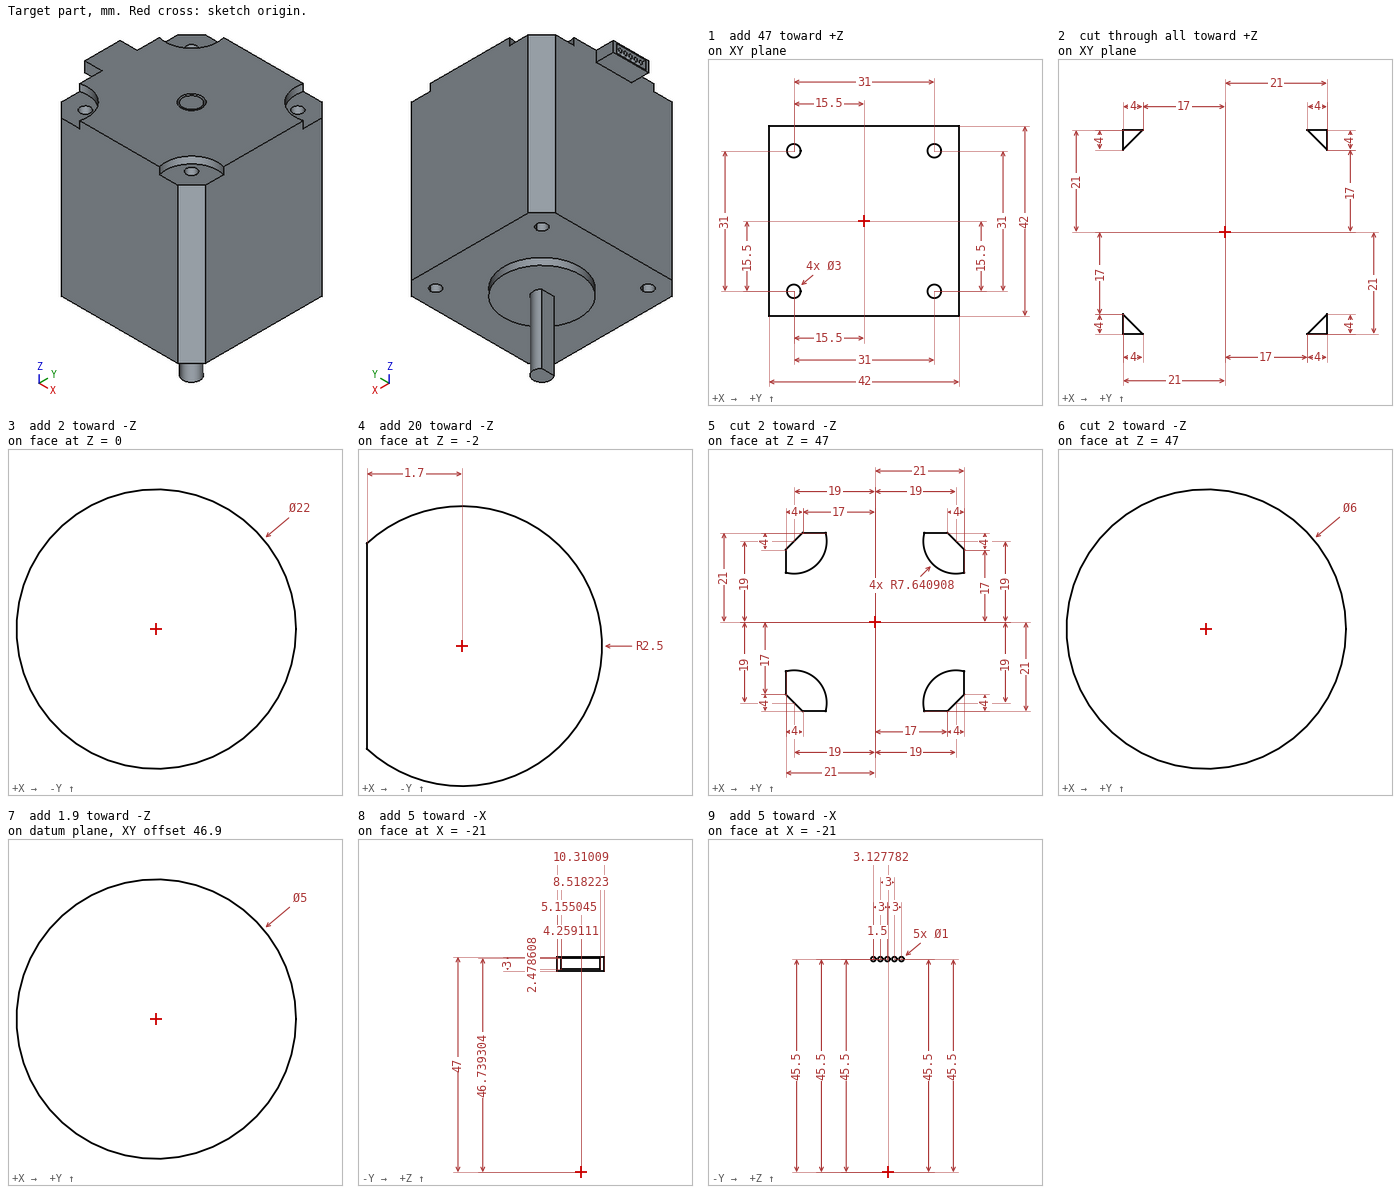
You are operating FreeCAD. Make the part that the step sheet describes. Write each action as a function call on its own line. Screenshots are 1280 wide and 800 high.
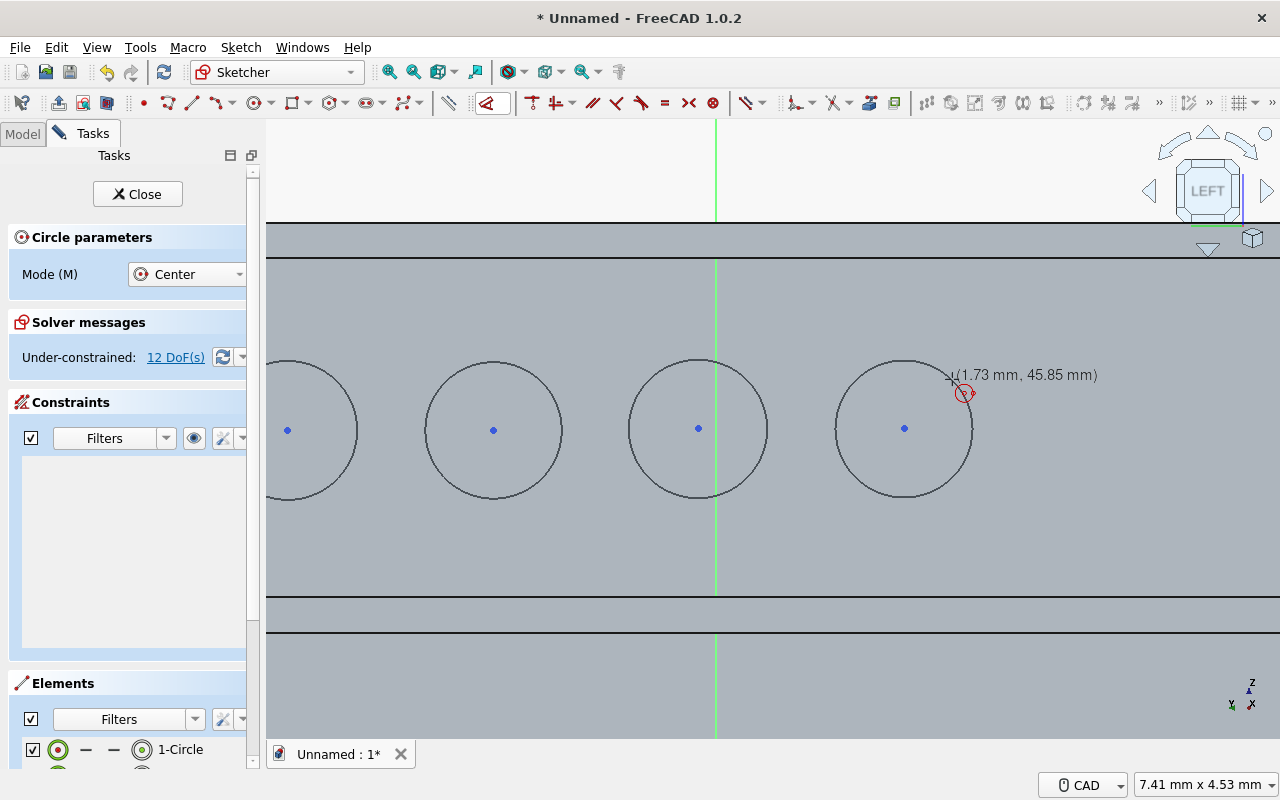
click(1109, 428)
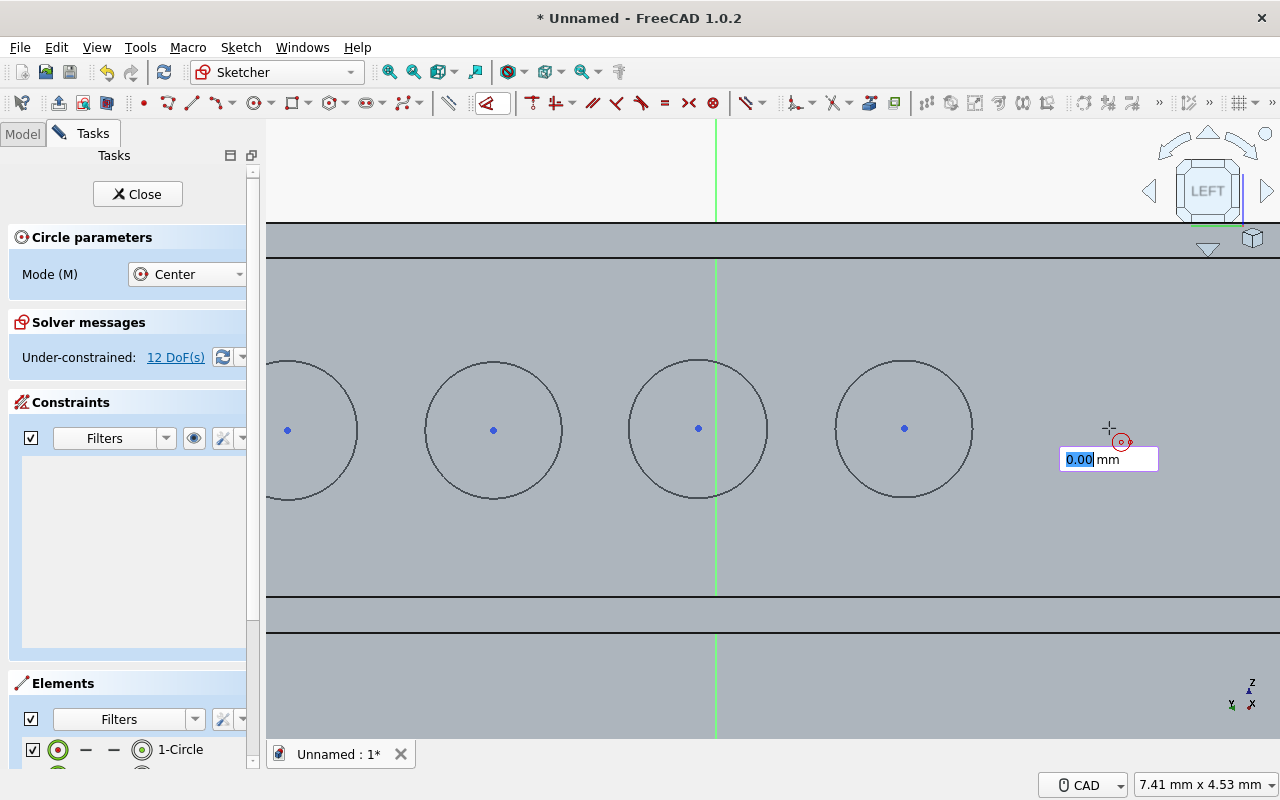
scroll(712, 431, down, 3)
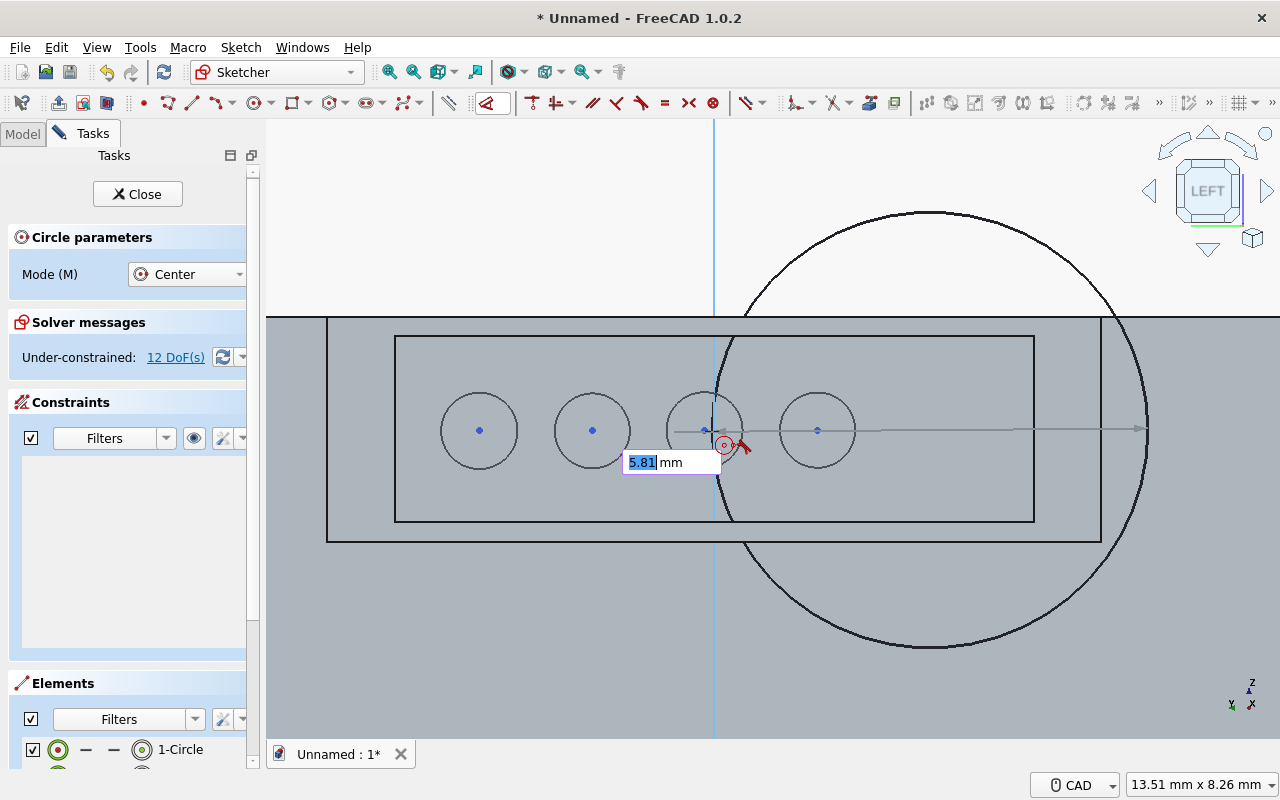
click(956, 403)
key(Escape)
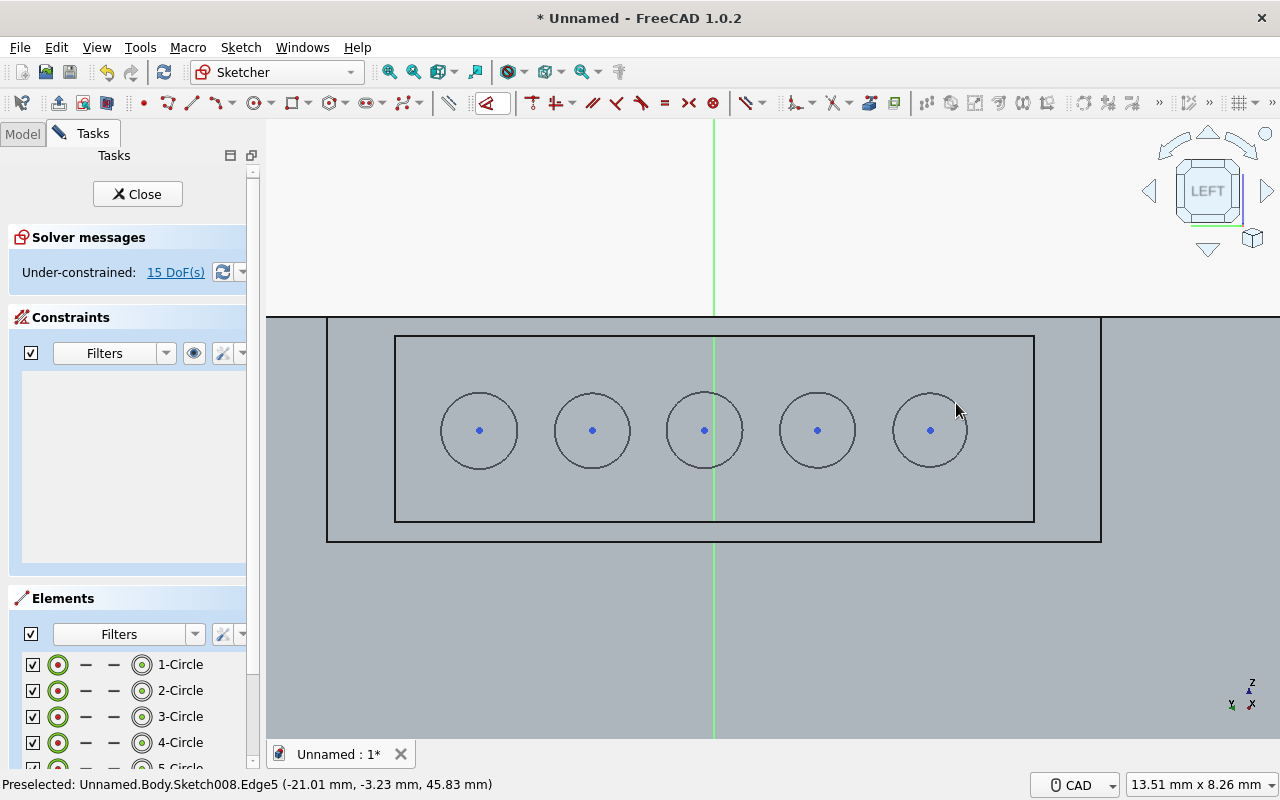
click(506, 404)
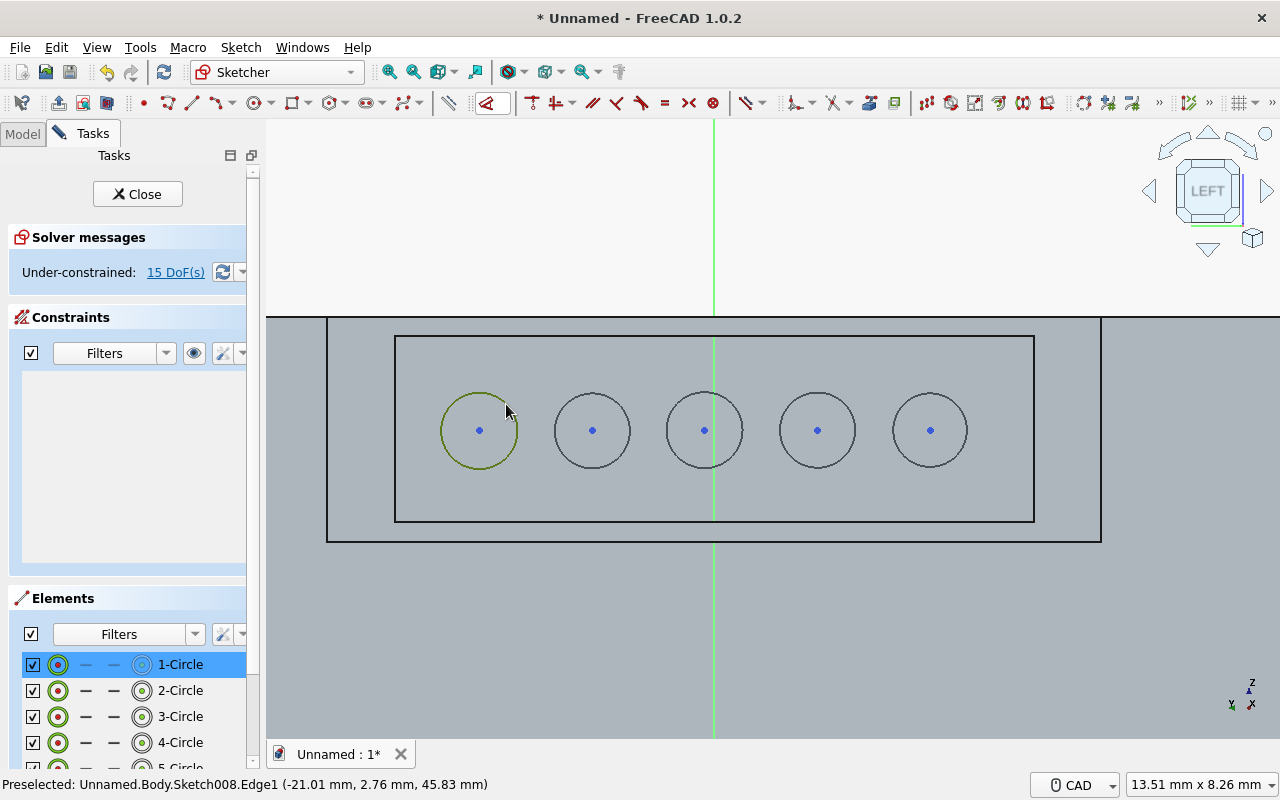
click(619, 404)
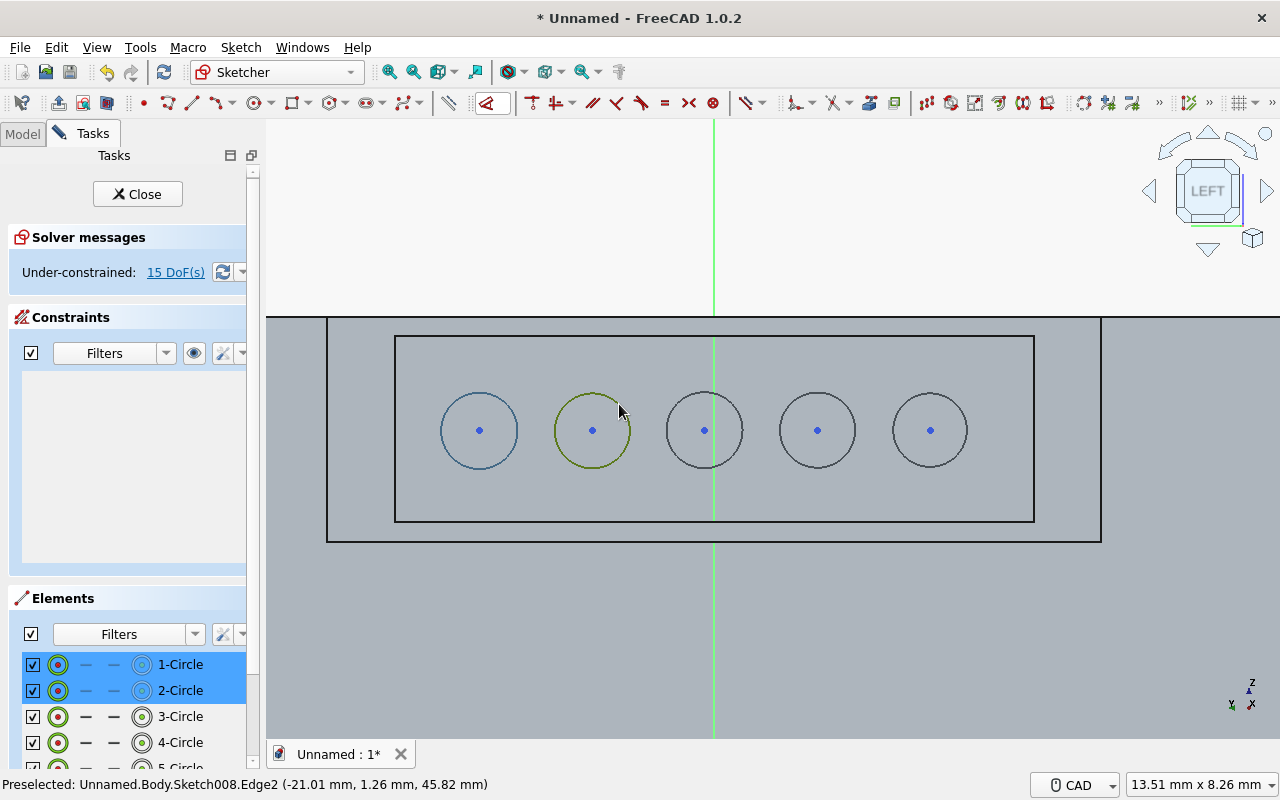
click(731, 403)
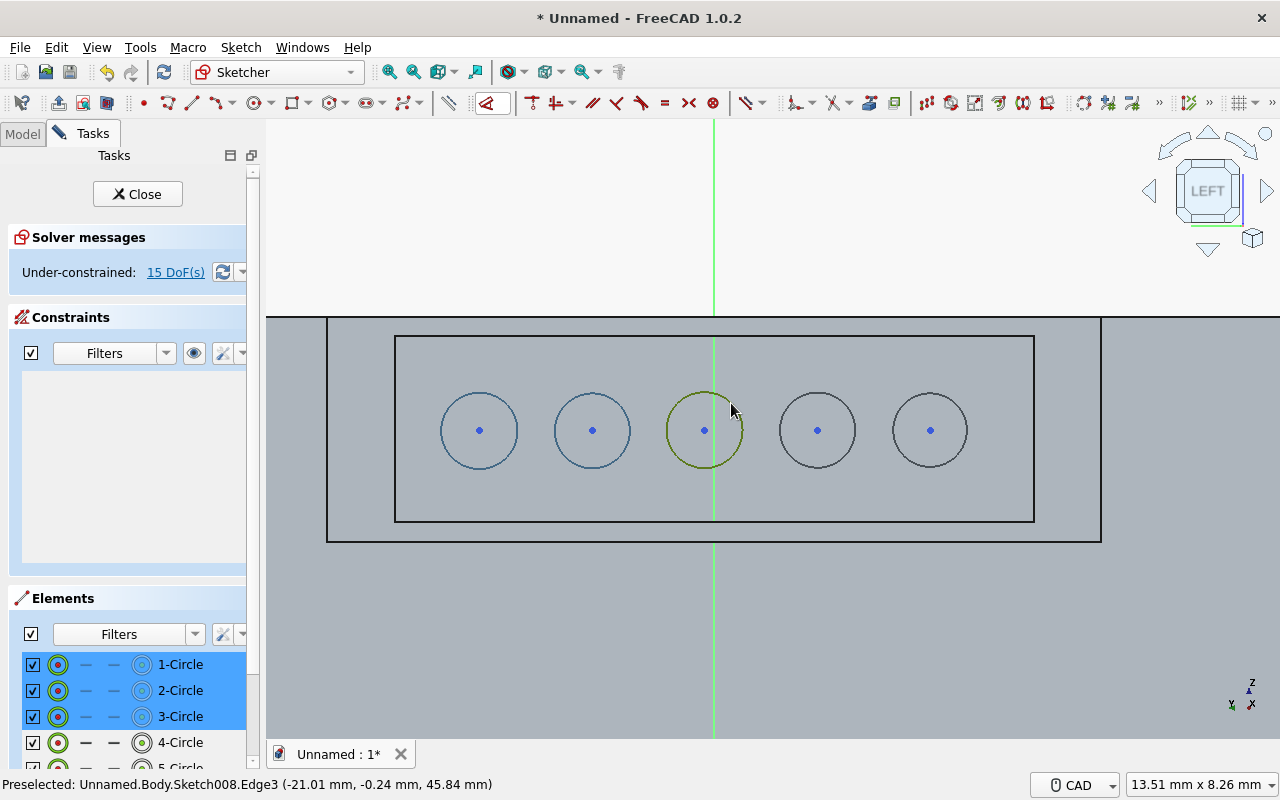
click(844, 403)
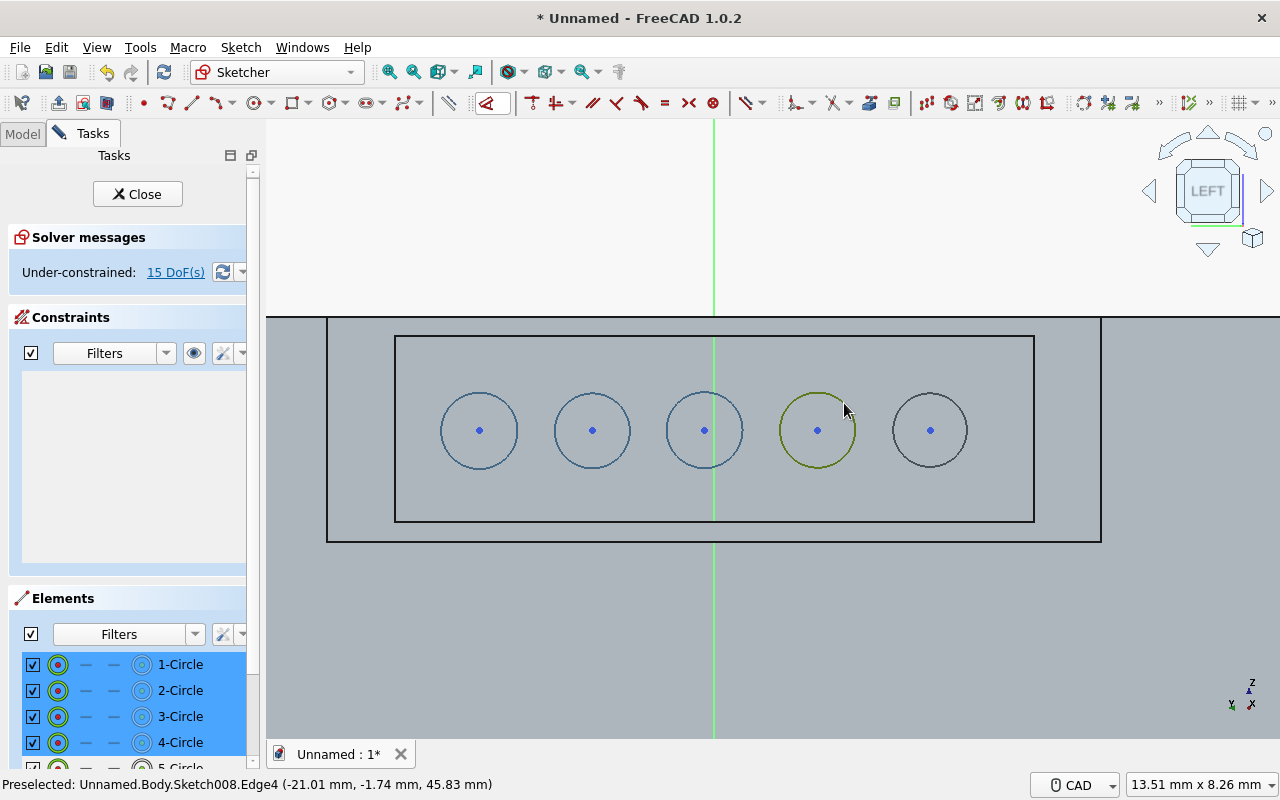
click(956, 404)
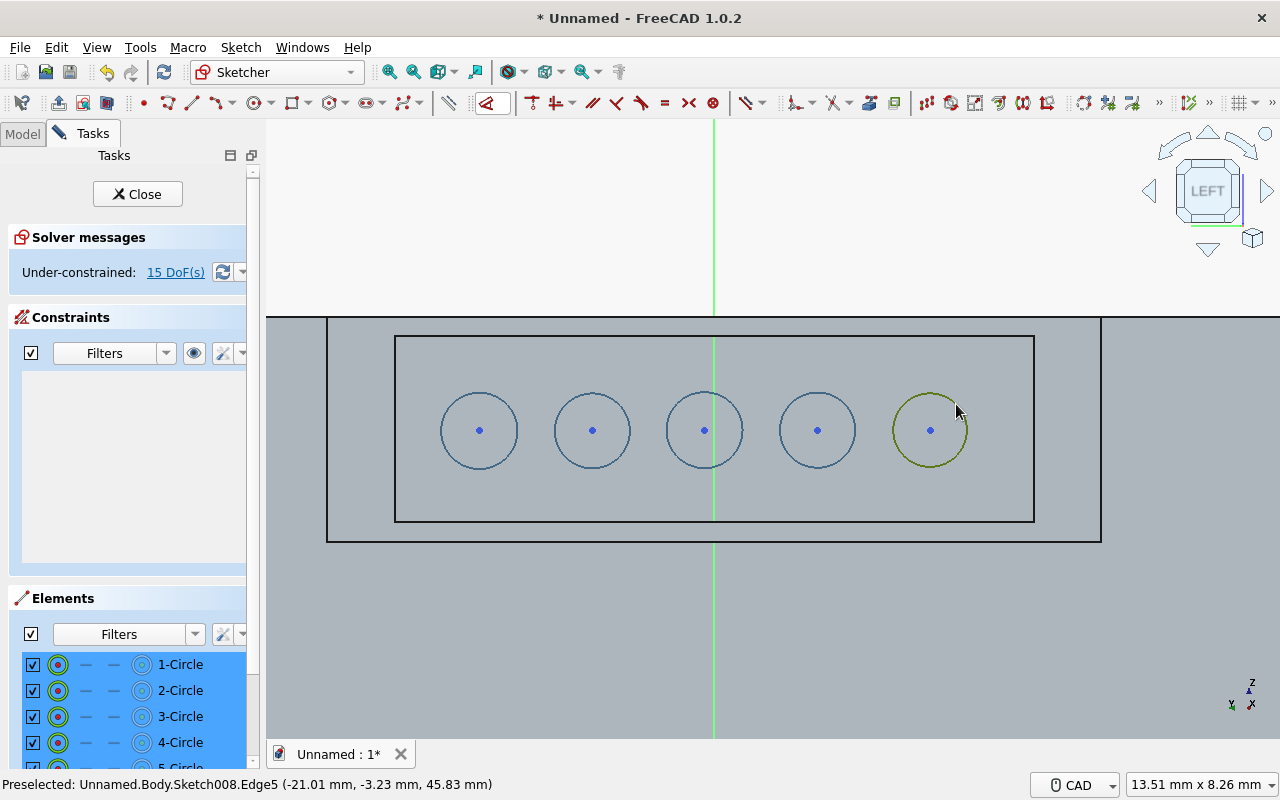
click(666, 104)